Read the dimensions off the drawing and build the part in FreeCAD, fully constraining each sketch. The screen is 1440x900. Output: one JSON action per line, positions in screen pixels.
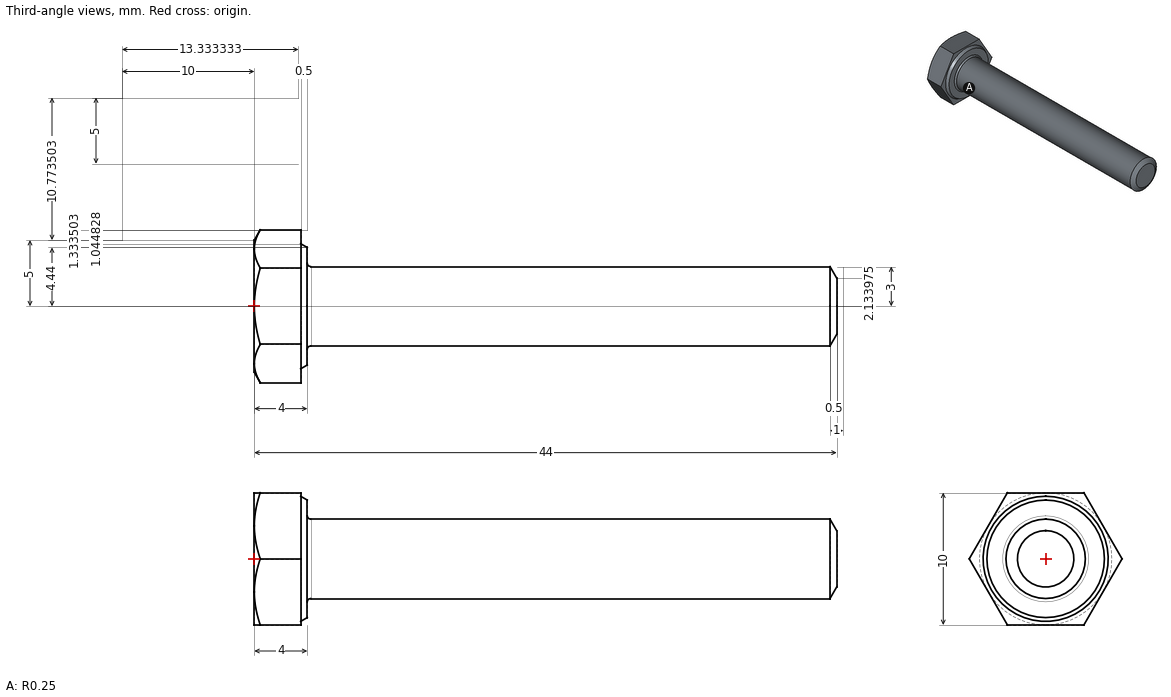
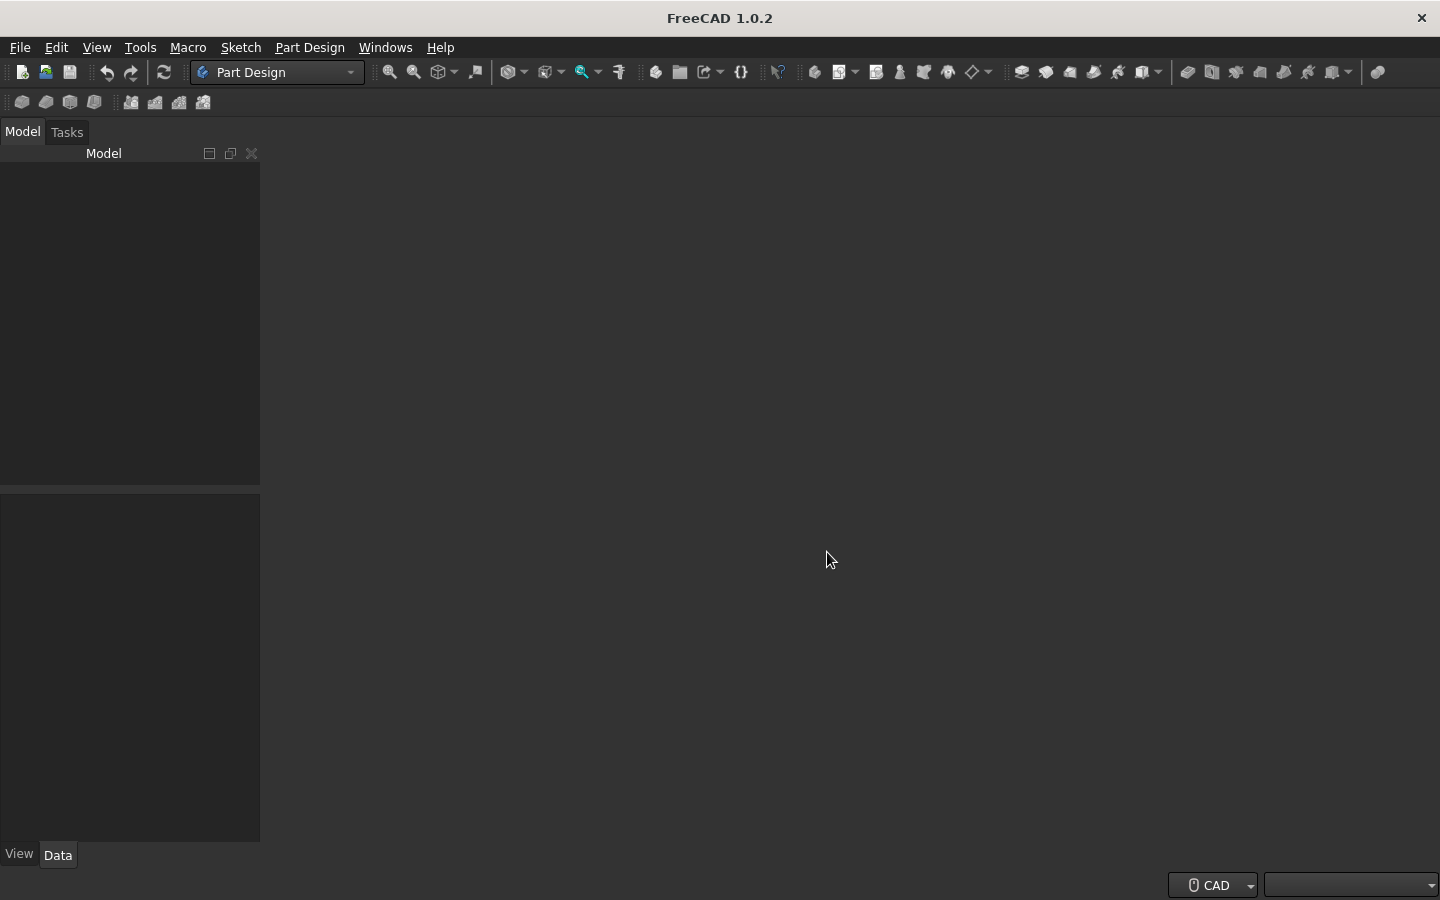
{"action": "left_click", "coordinate": [22, 72]}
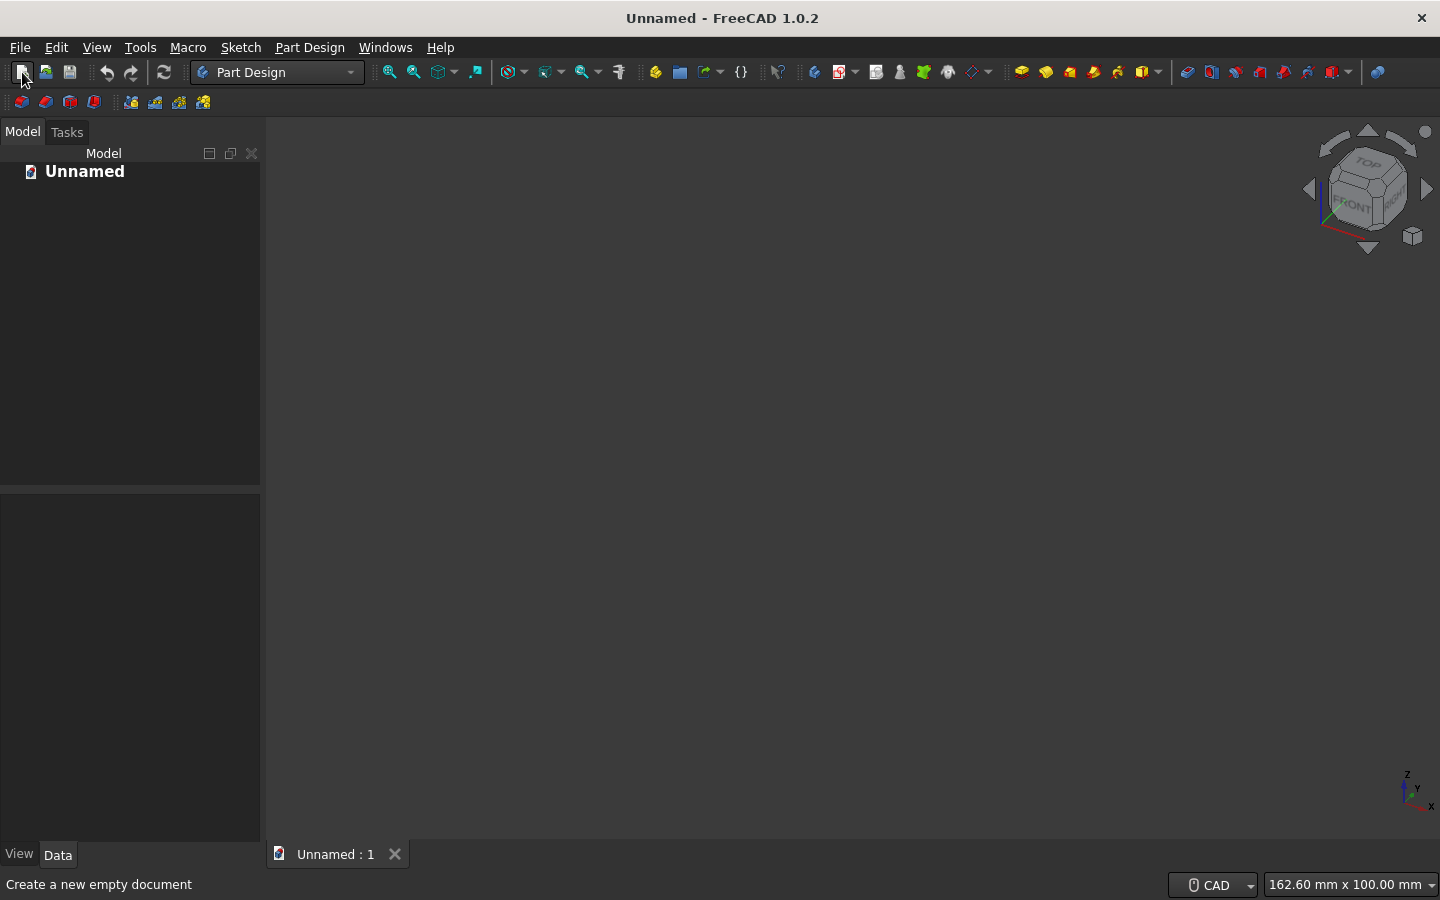
{"action": "left_click", "coordinate": [840, 72]}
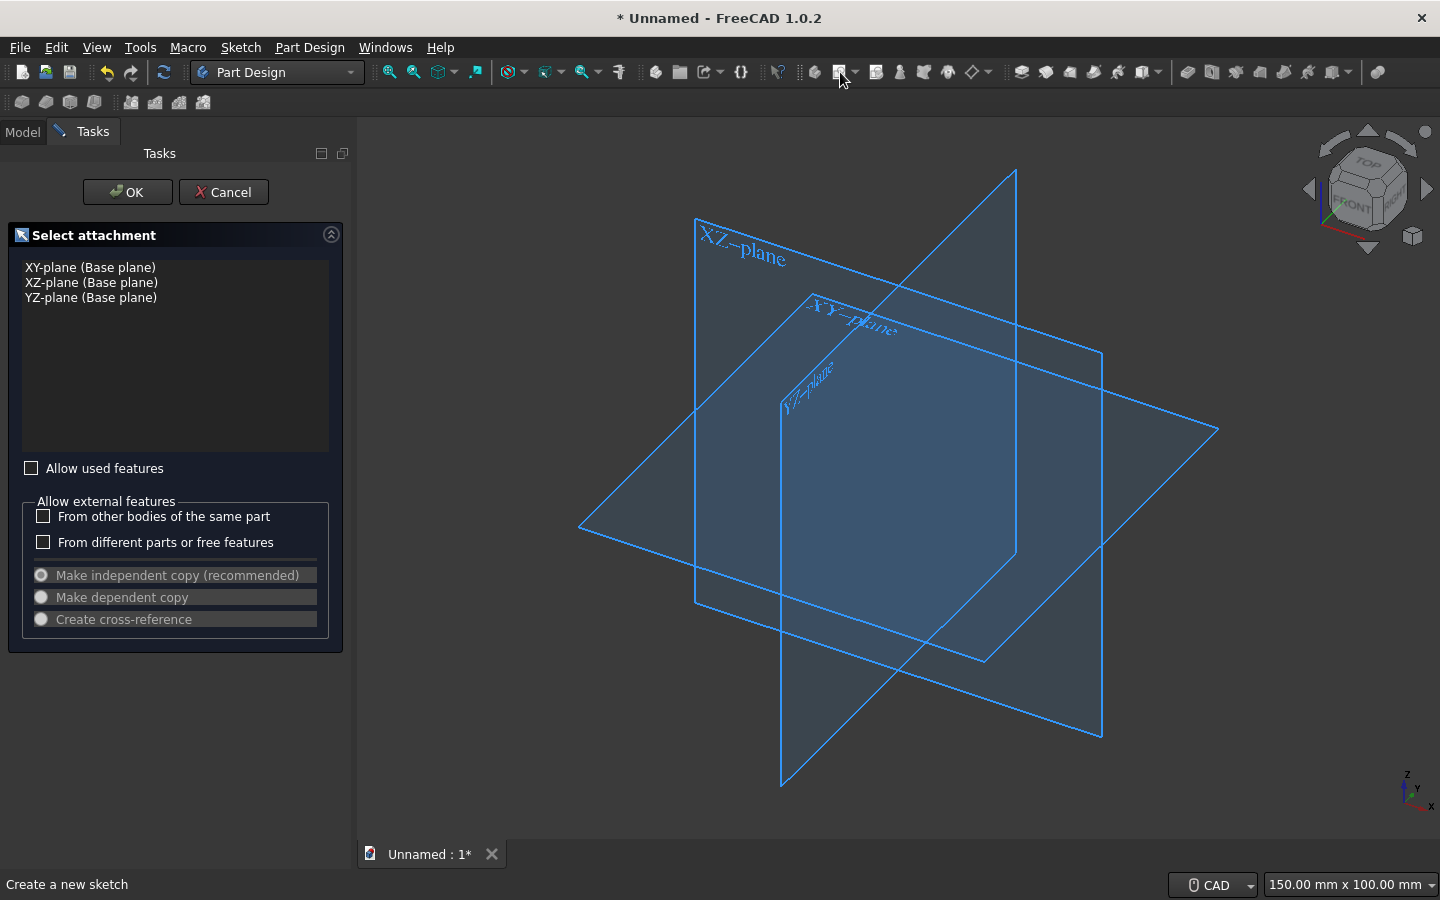
{"action": "left_click", "coordinate": [82, 298]}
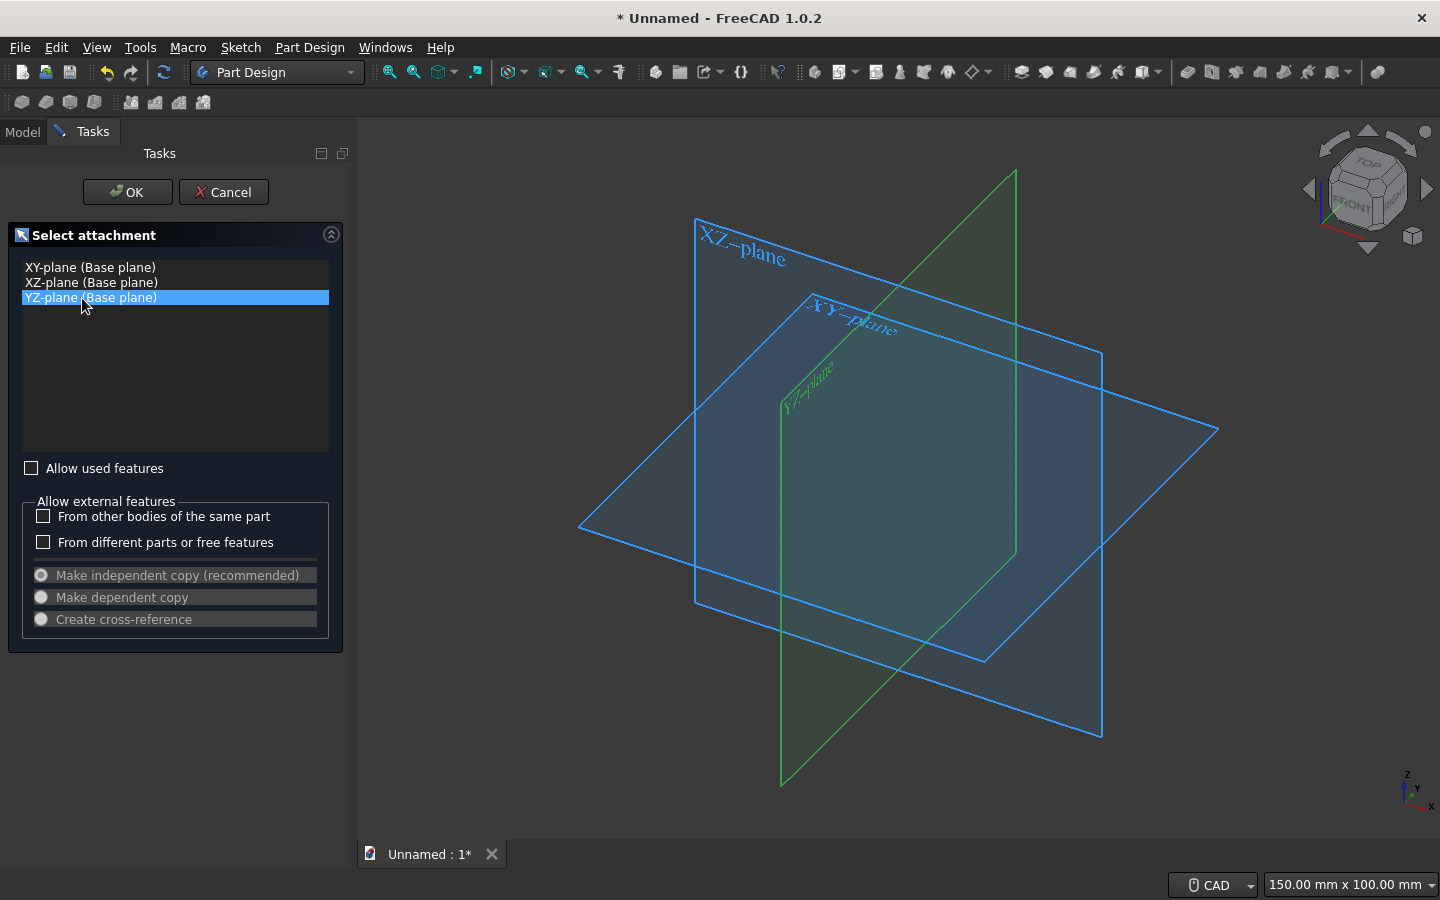
{"action": "left_click", "coordinate": [128, 192]}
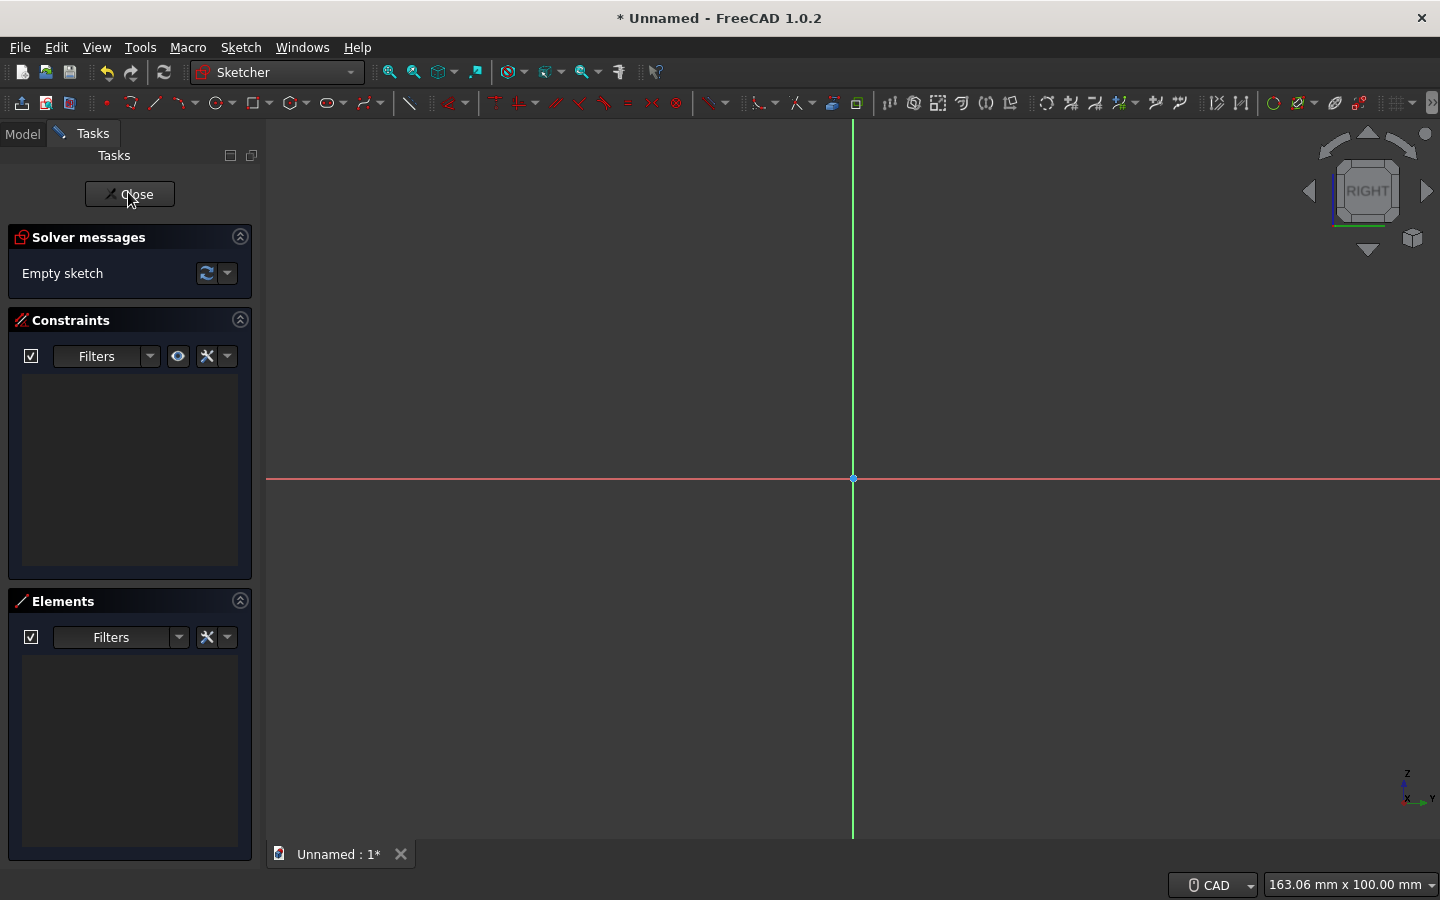
{"action": "scroll", "coordinate": [867, 479], "scroll_direction": "up", "scroll_amount": 9}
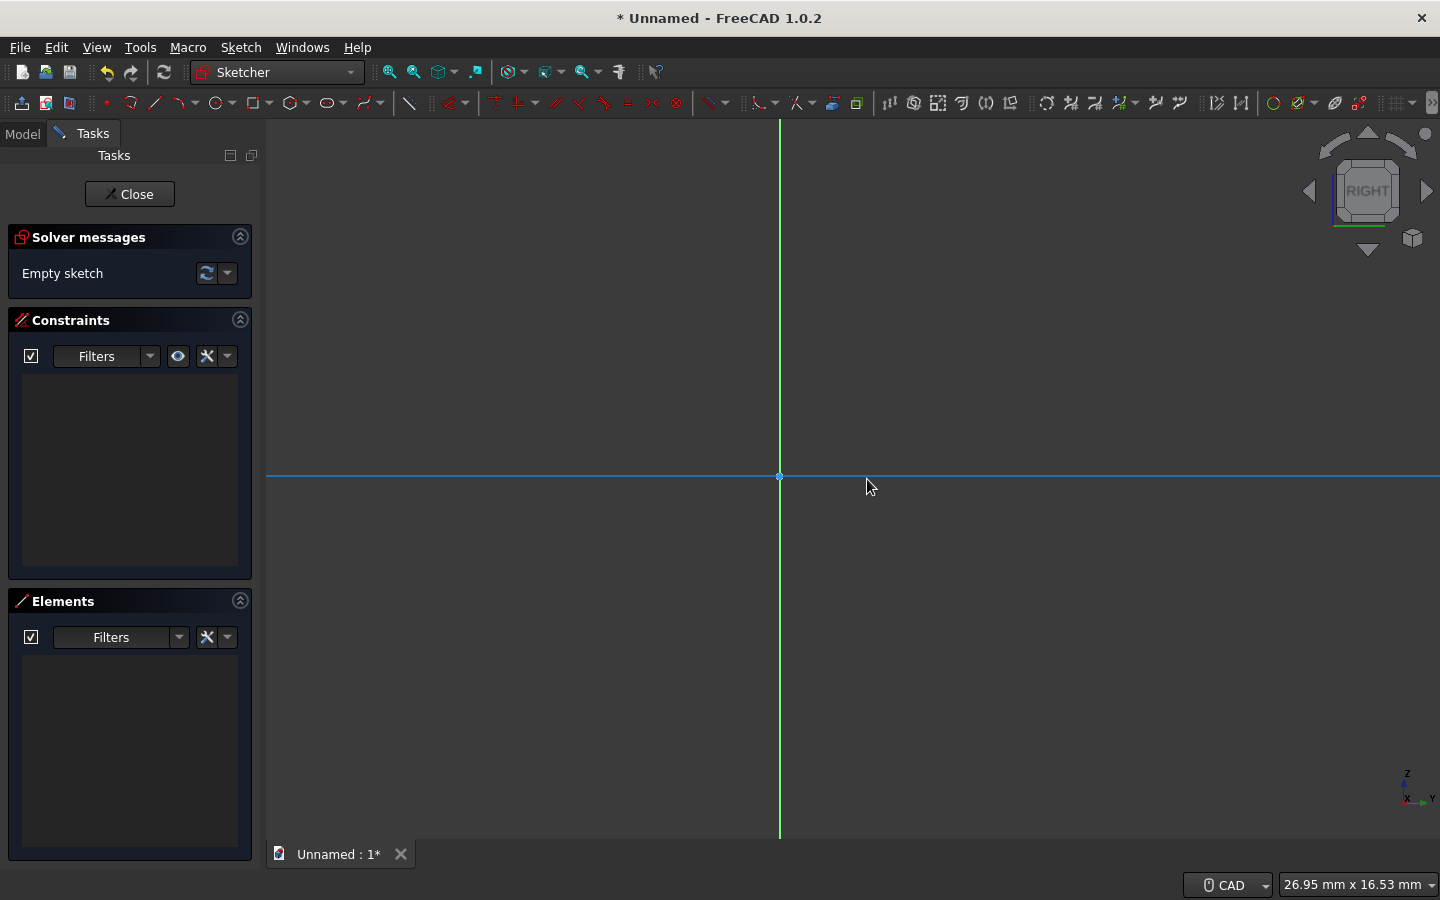
{"action": "left_click", "coordinate": [290, 104]}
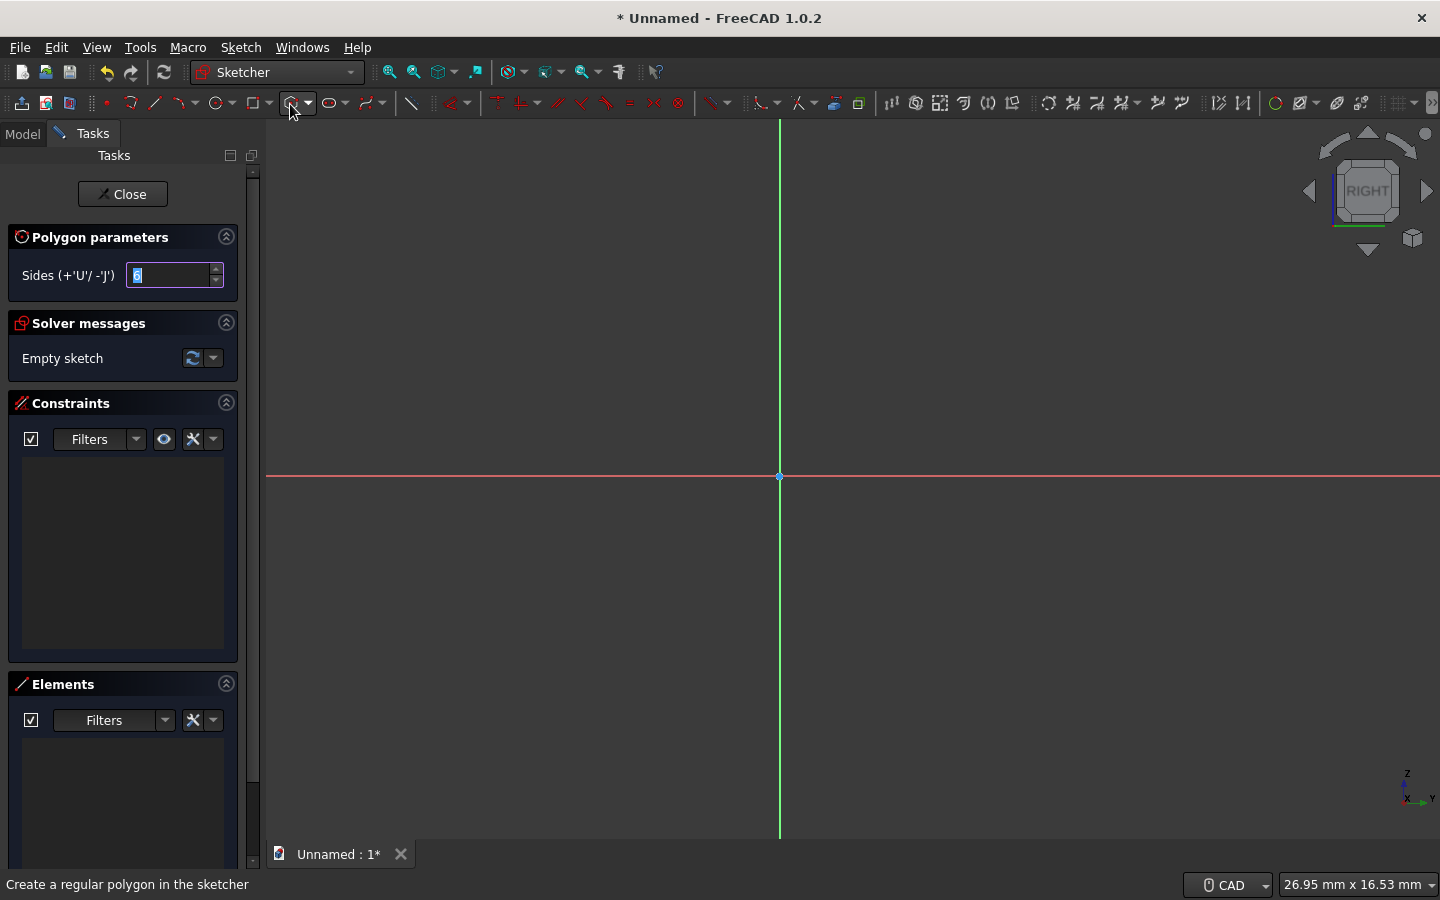
{"action": "left_click", "coordinate": [780, 476]}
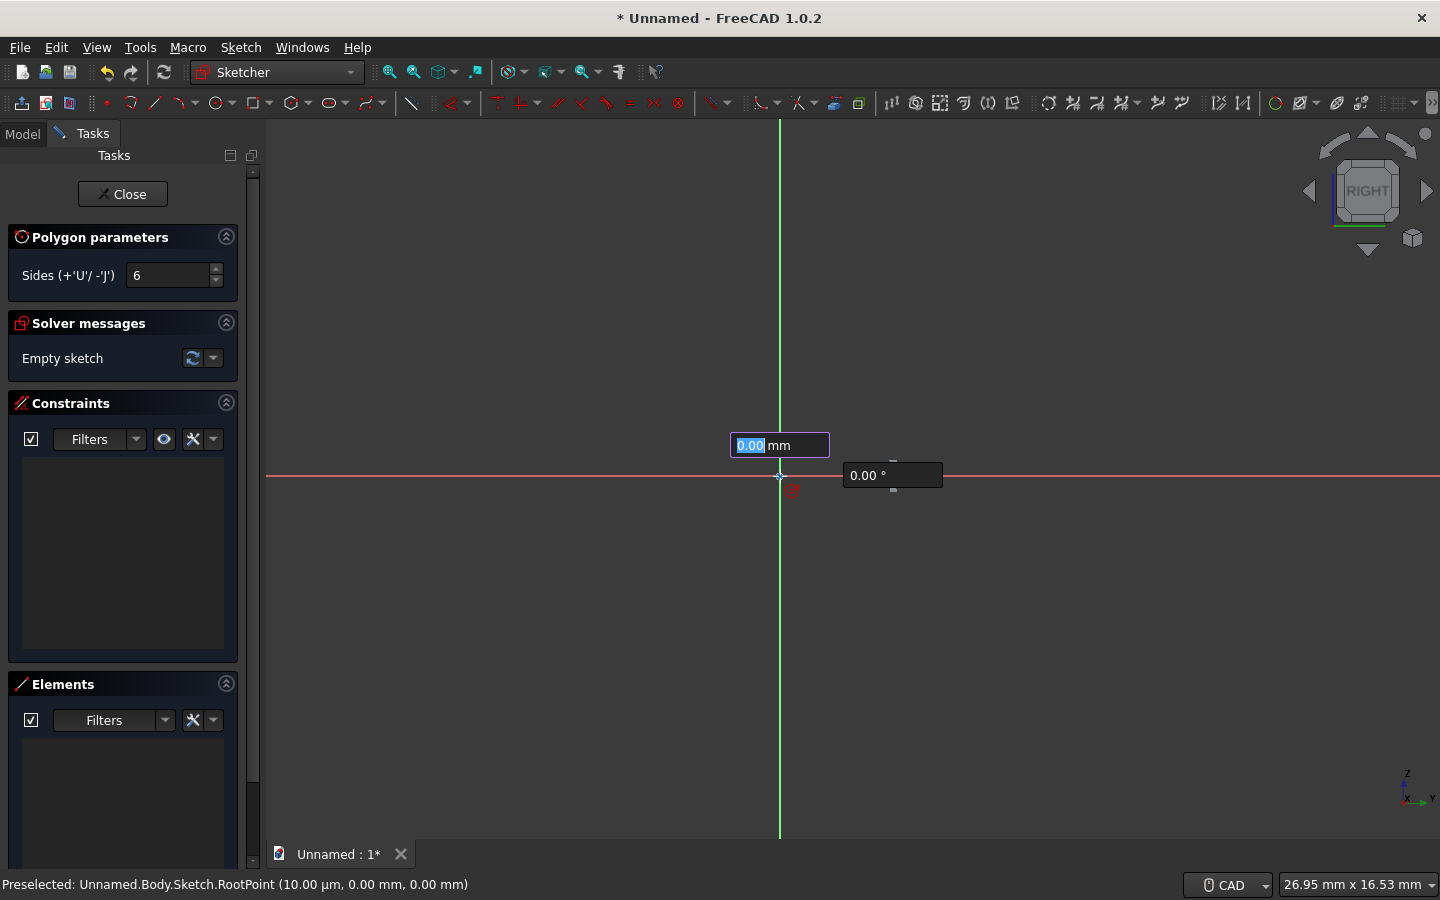
{"action": "left_click", "coordinate": [1031, 476]}
{"action": "key", "text": "Escape"}